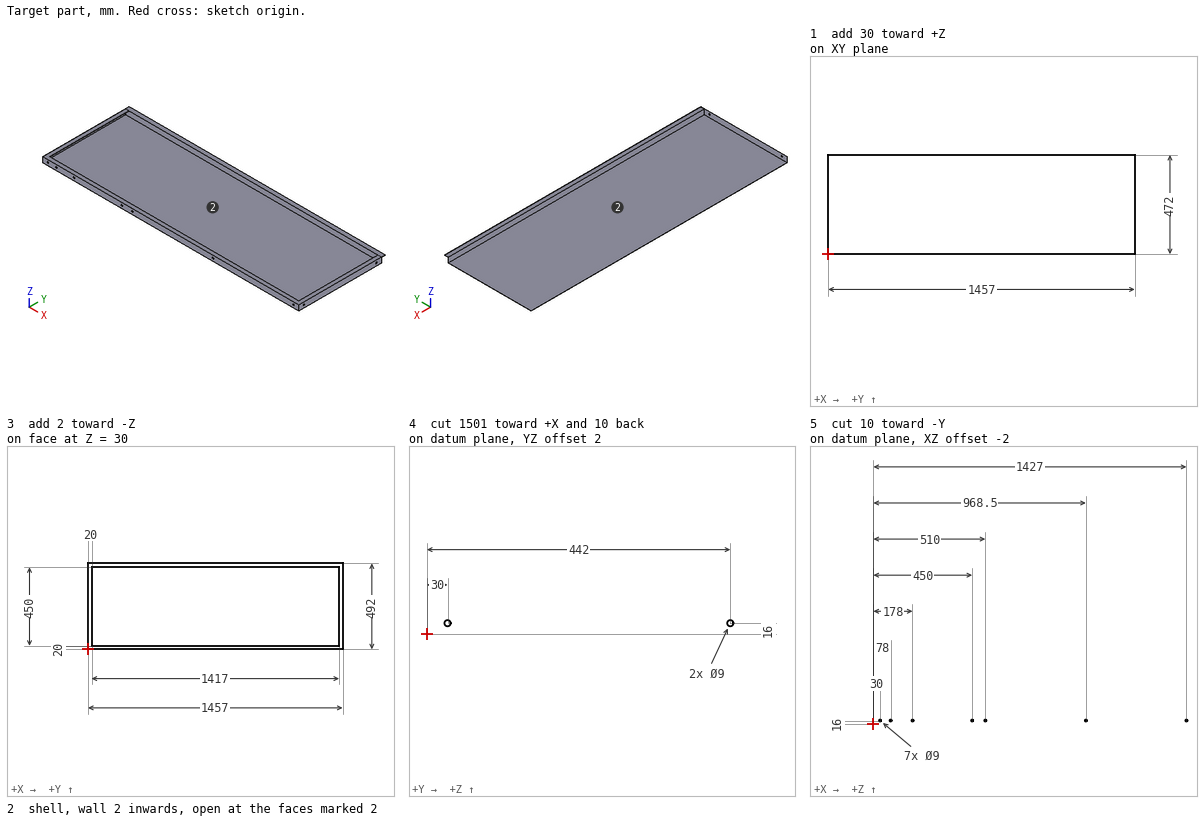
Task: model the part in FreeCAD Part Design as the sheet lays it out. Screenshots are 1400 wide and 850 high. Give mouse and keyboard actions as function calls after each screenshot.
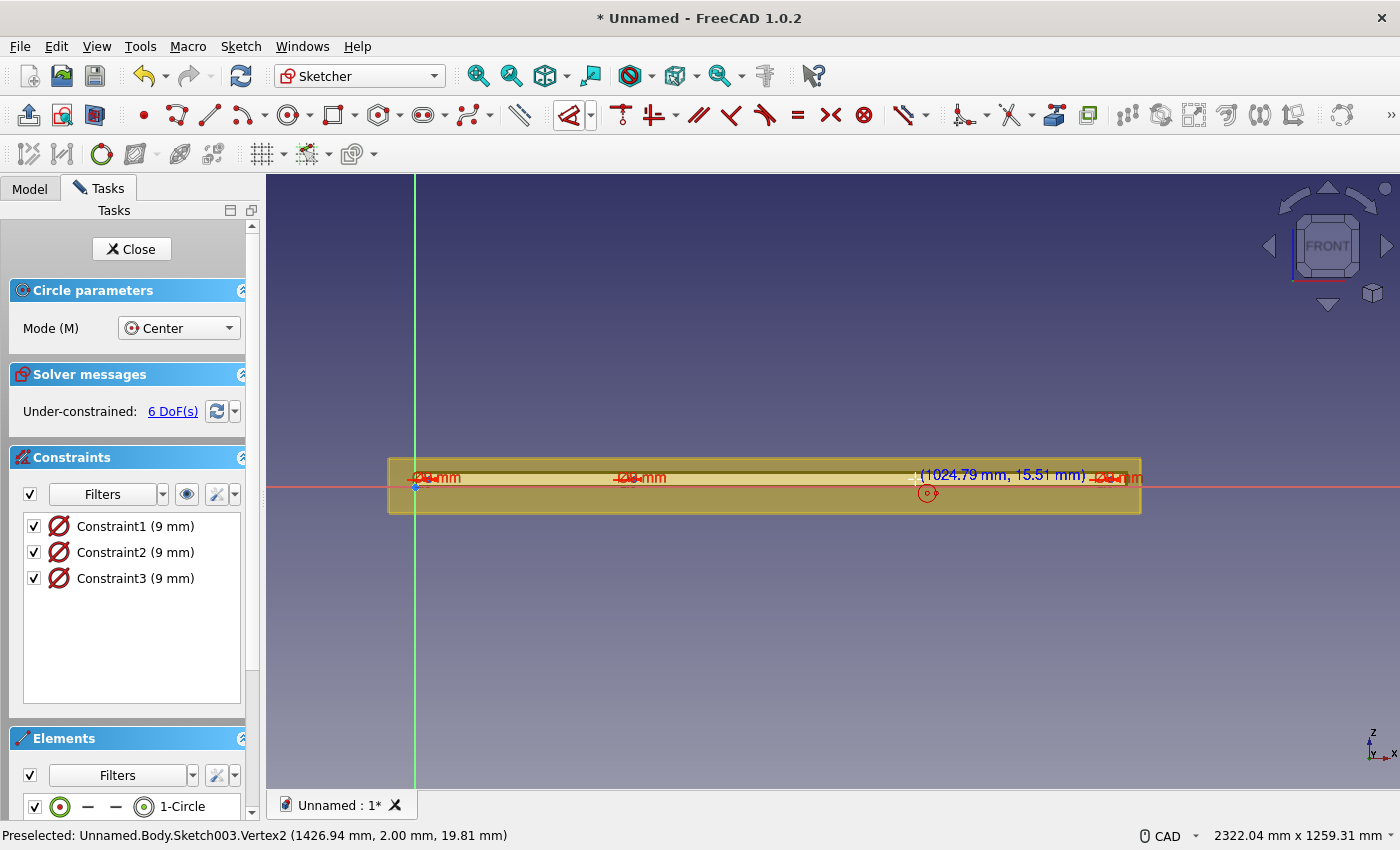
scroll(888, 479, up, 4)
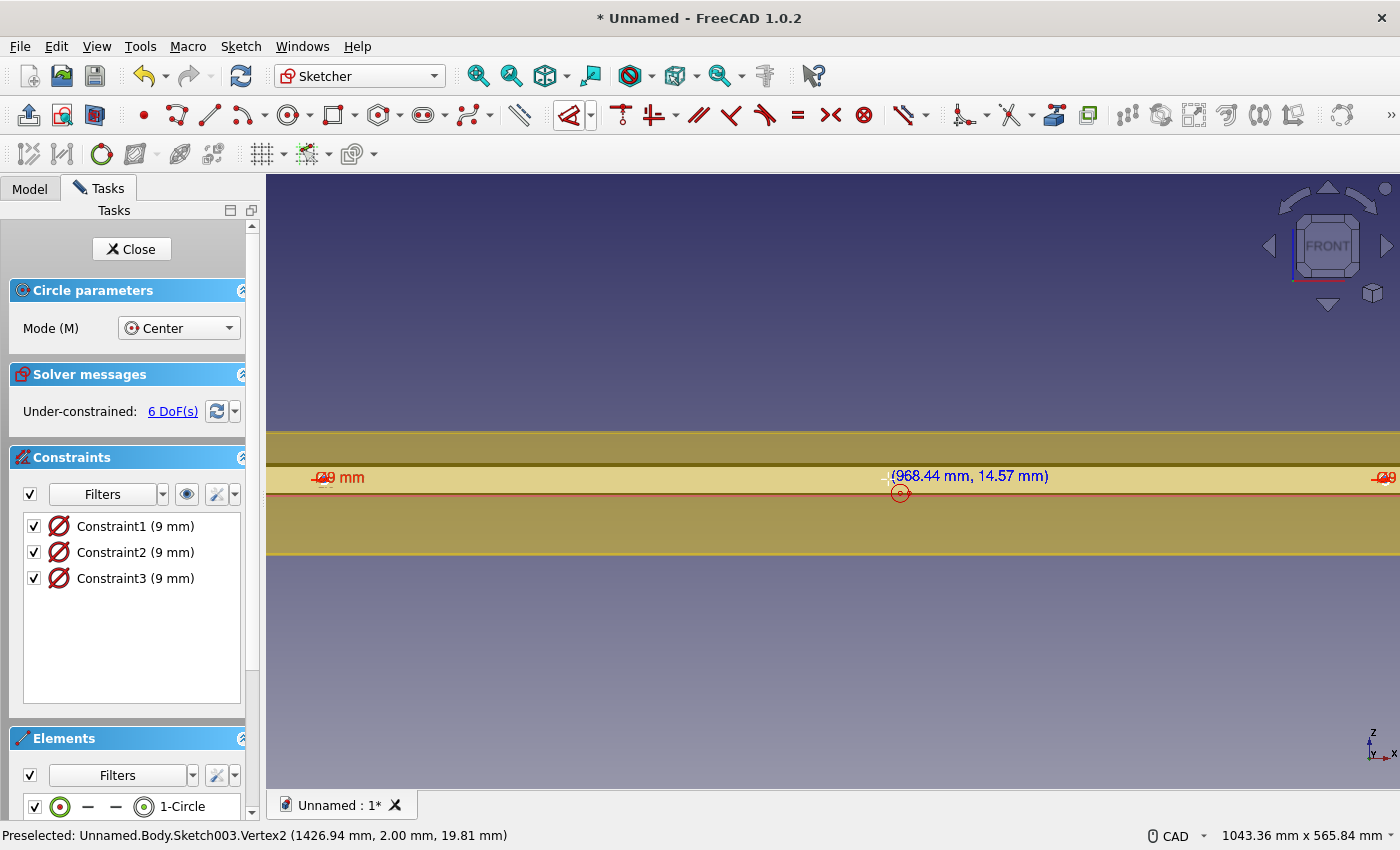
click(887, 479)
move(891, 476)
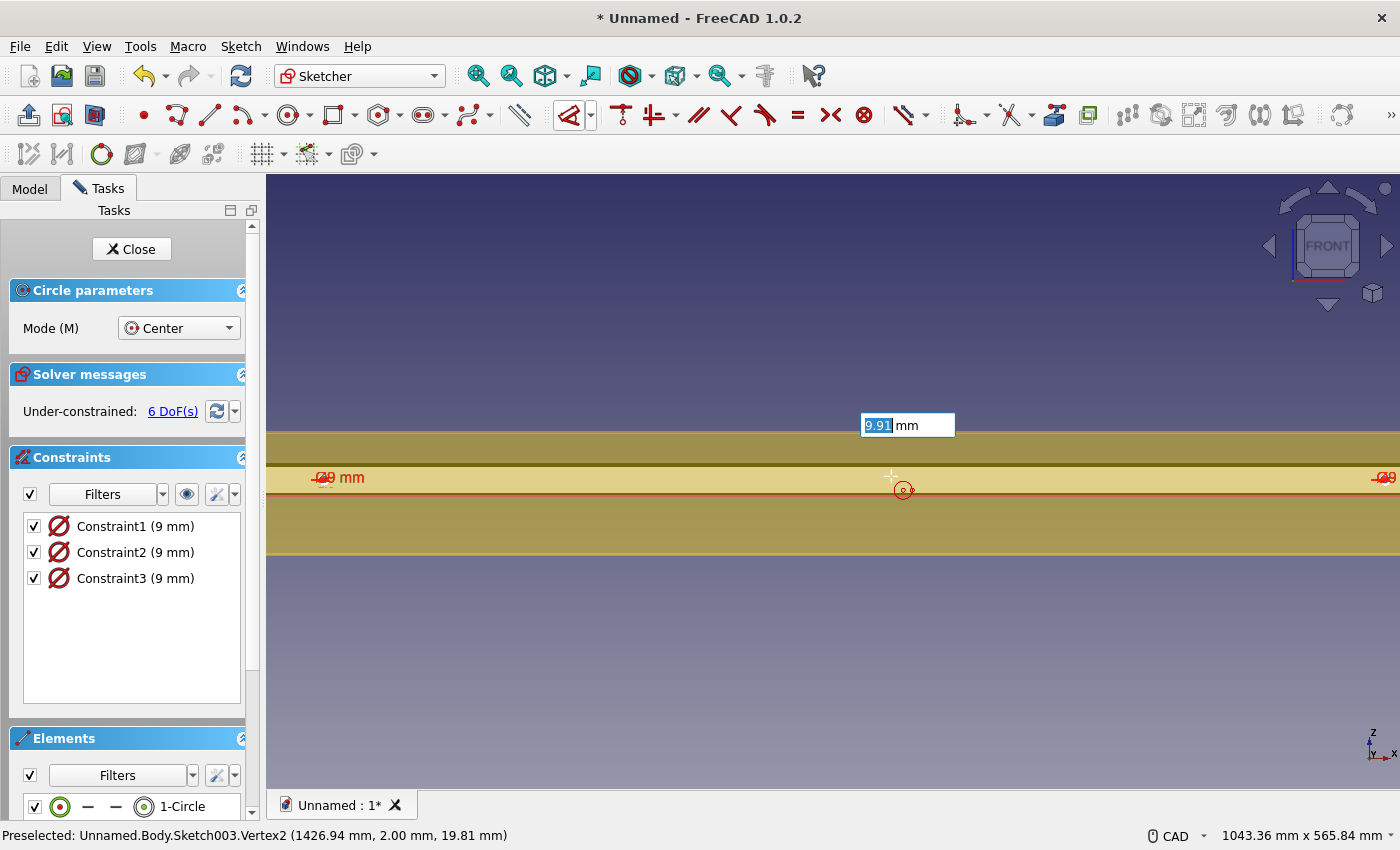
text(9)
key(Return)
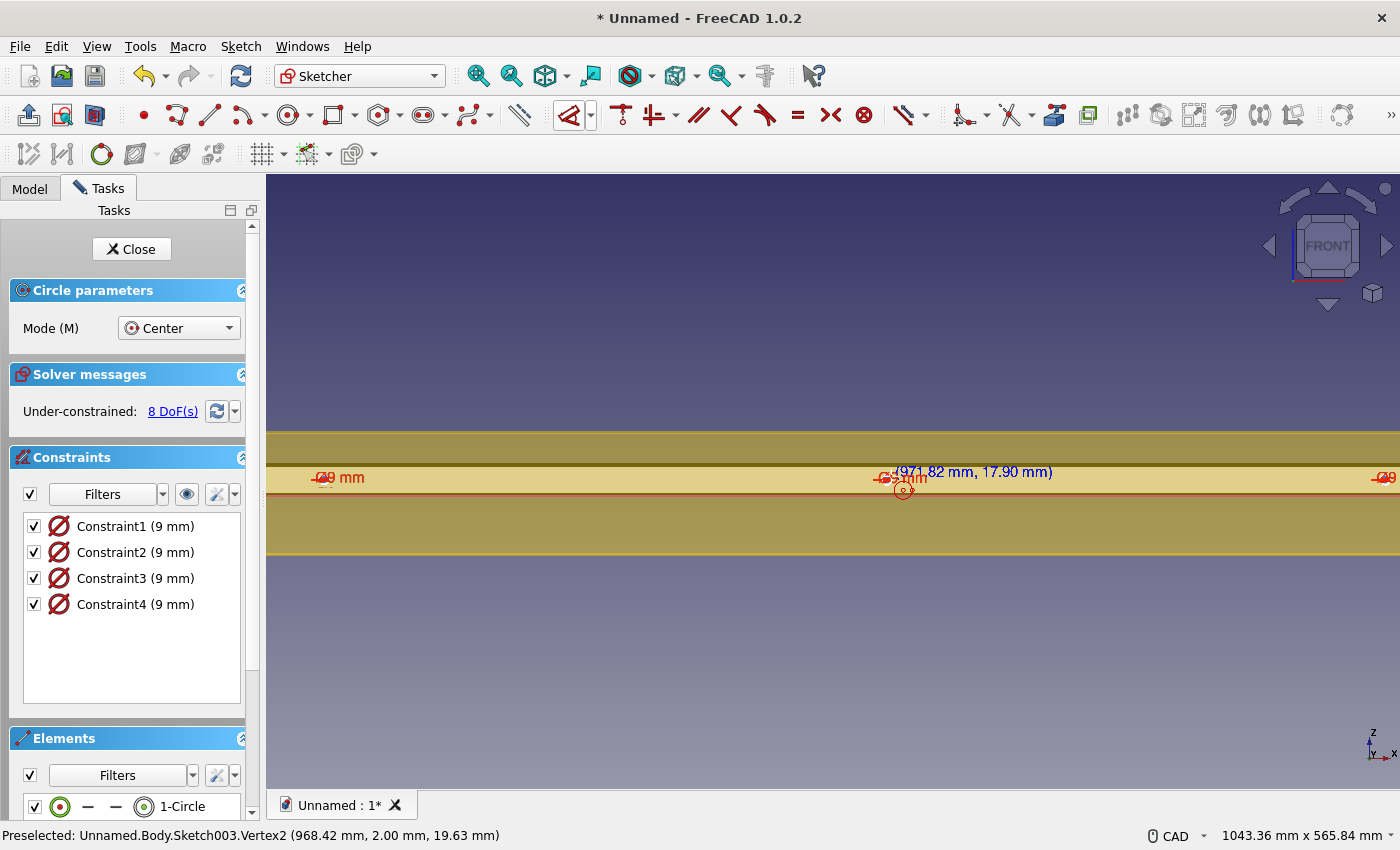
scroll(389, 479, up, 8)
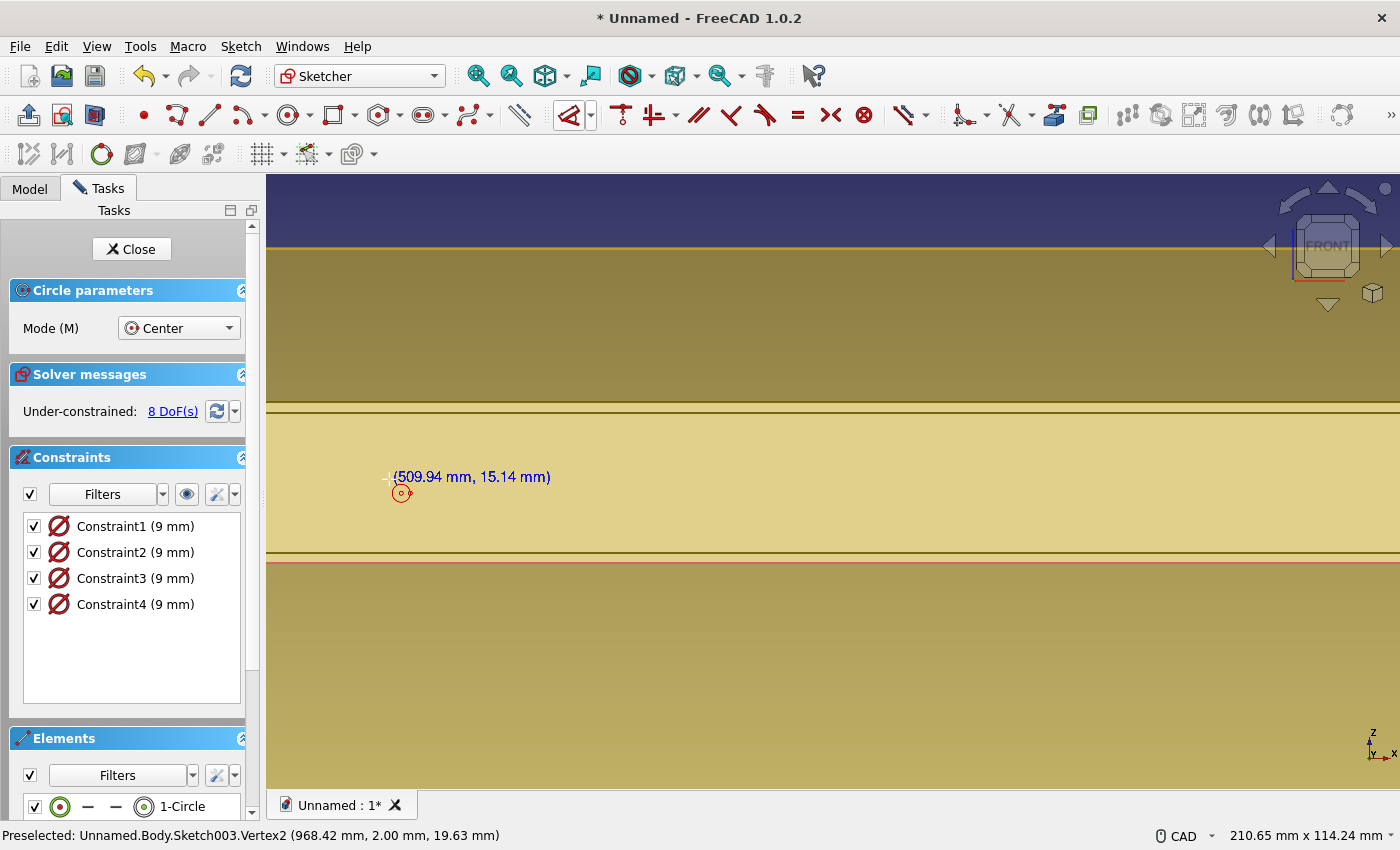
scroll(691, 479, down, 12)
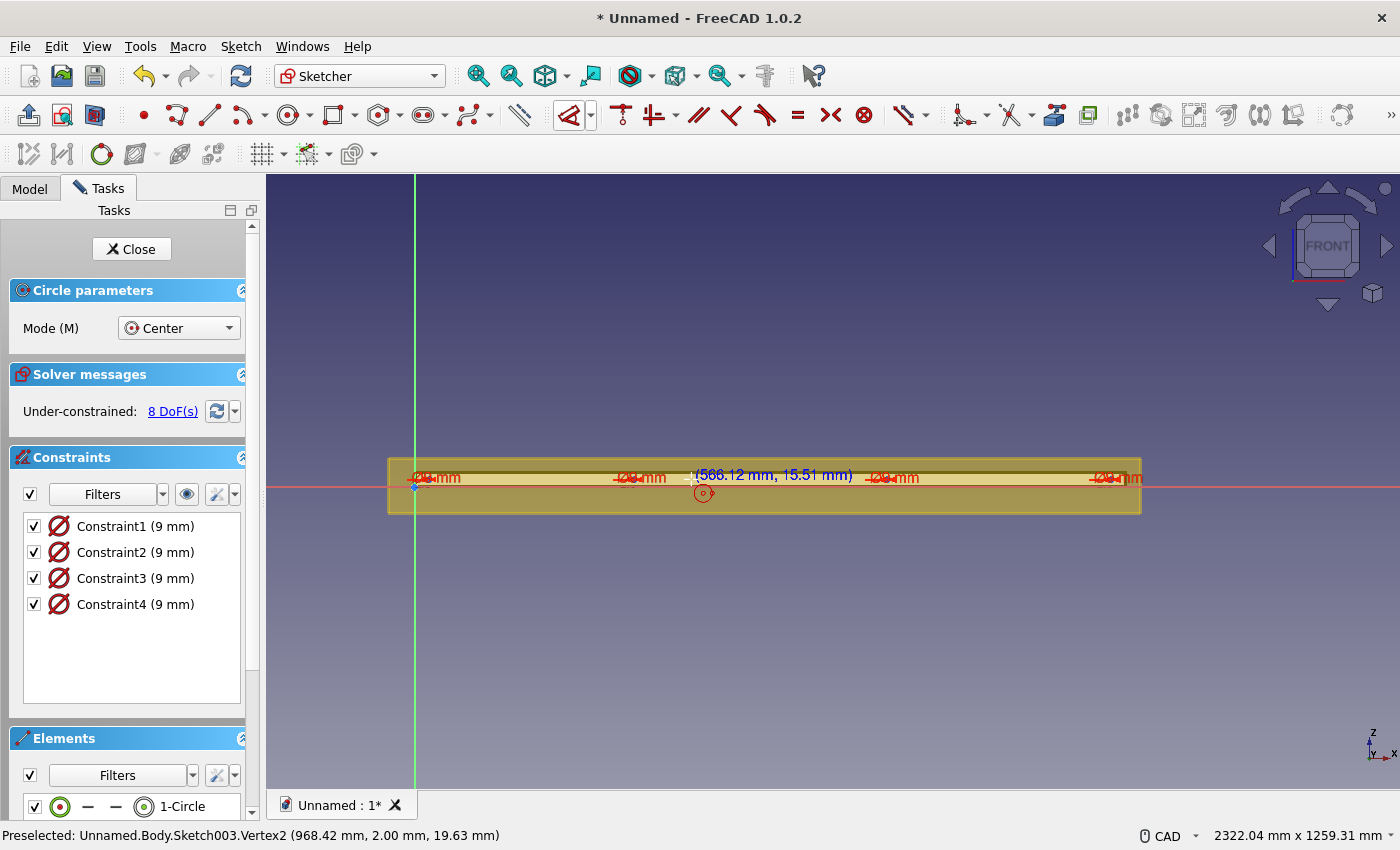
scroll(664, 479, up, 4)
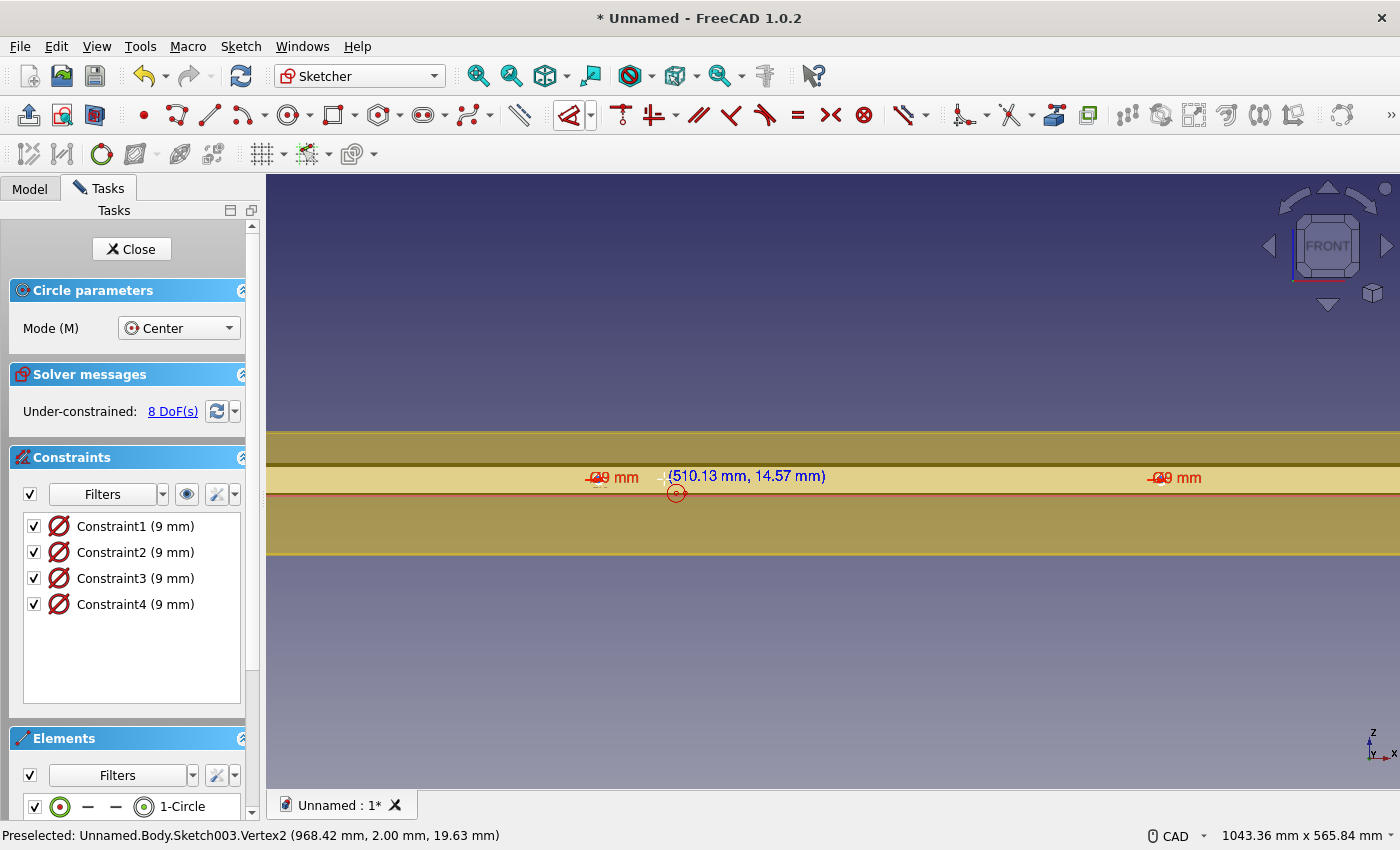
click(663, 479)
move(667, 476)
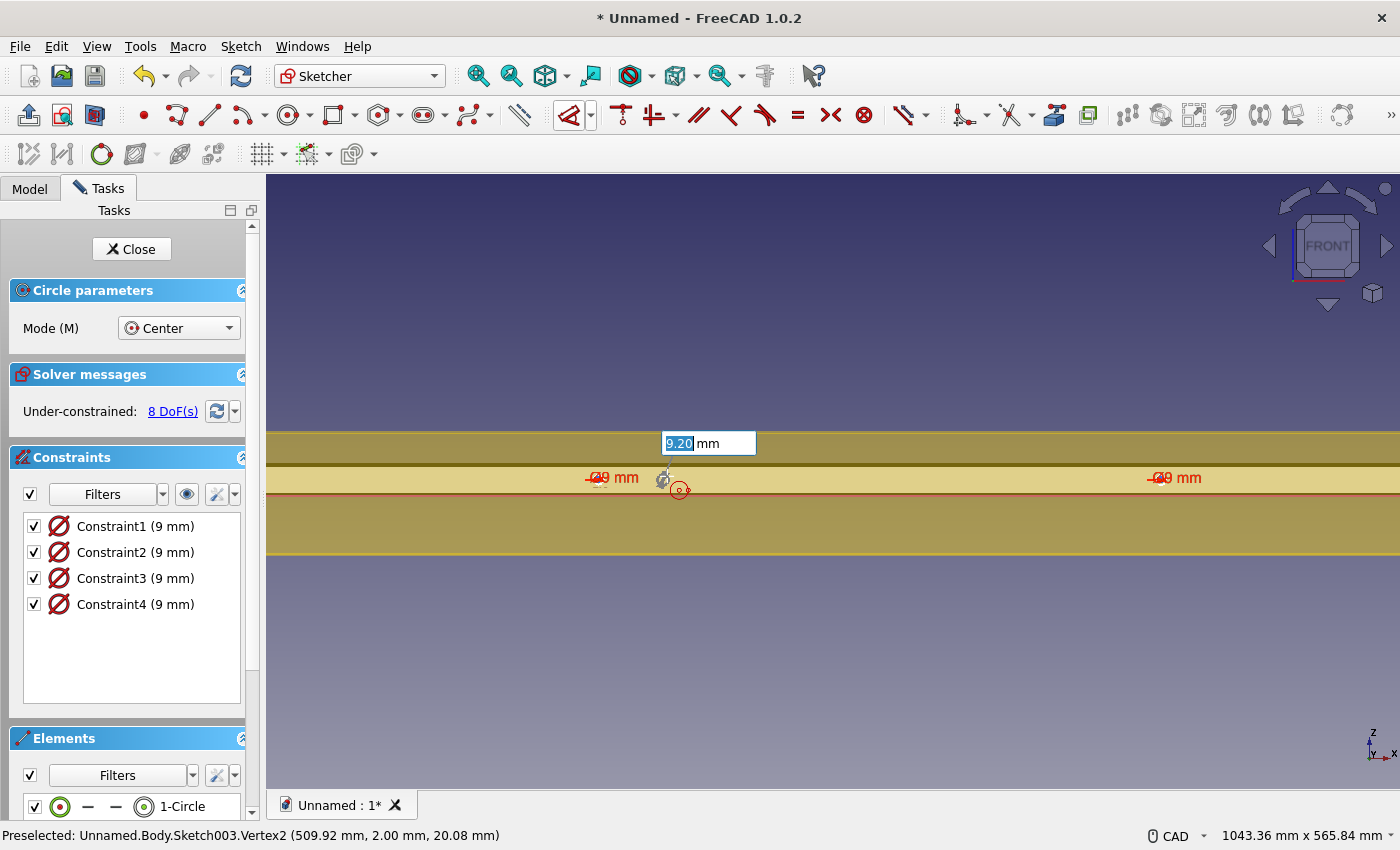
text(9)
key(Return)